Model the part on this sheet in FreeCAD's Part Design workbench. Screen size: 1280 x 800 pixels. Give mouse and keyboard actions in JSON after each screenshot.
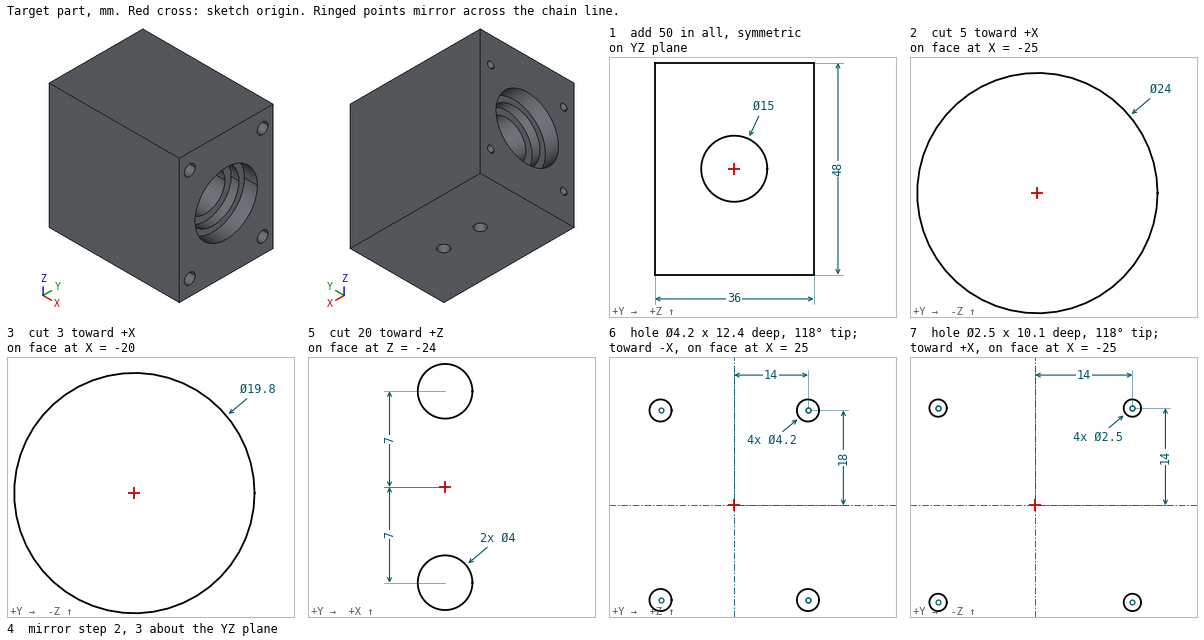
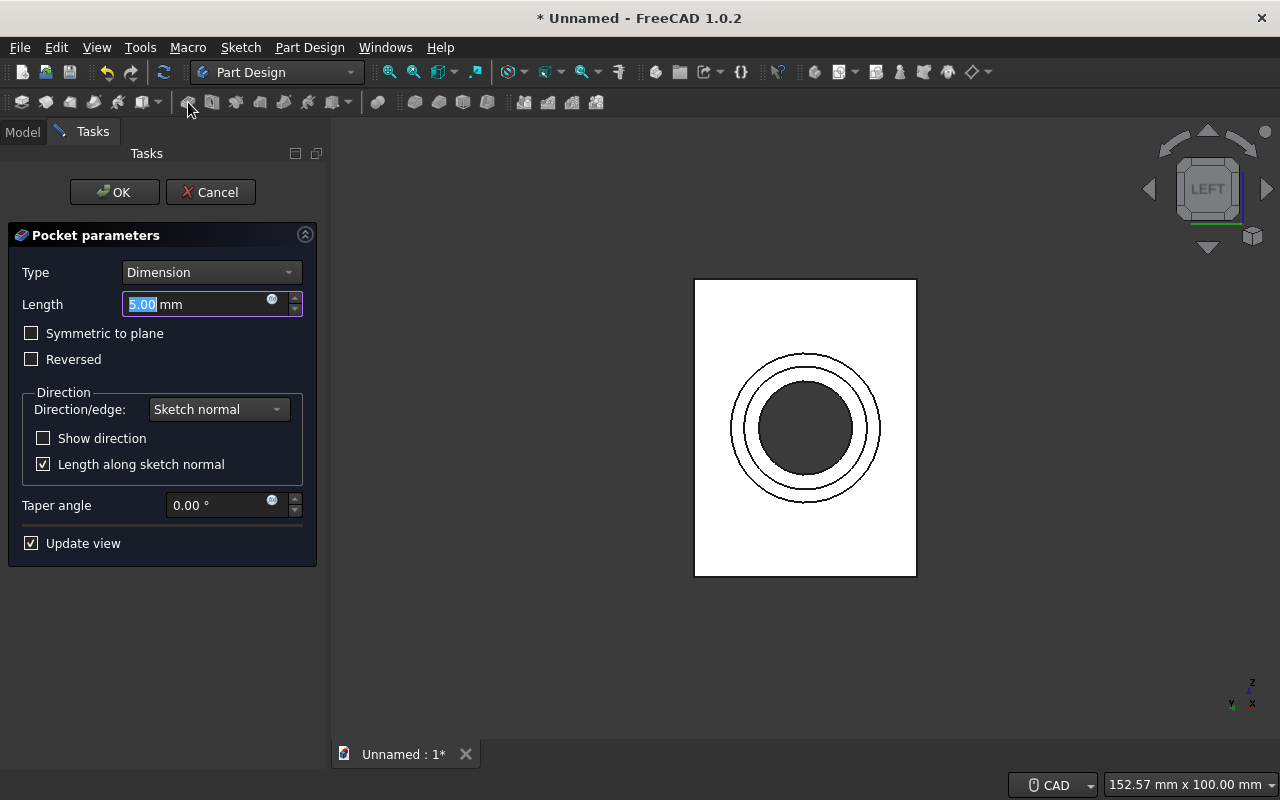
{"action": "type", "text": "3"}
{"action": "key", "text": "Tab"}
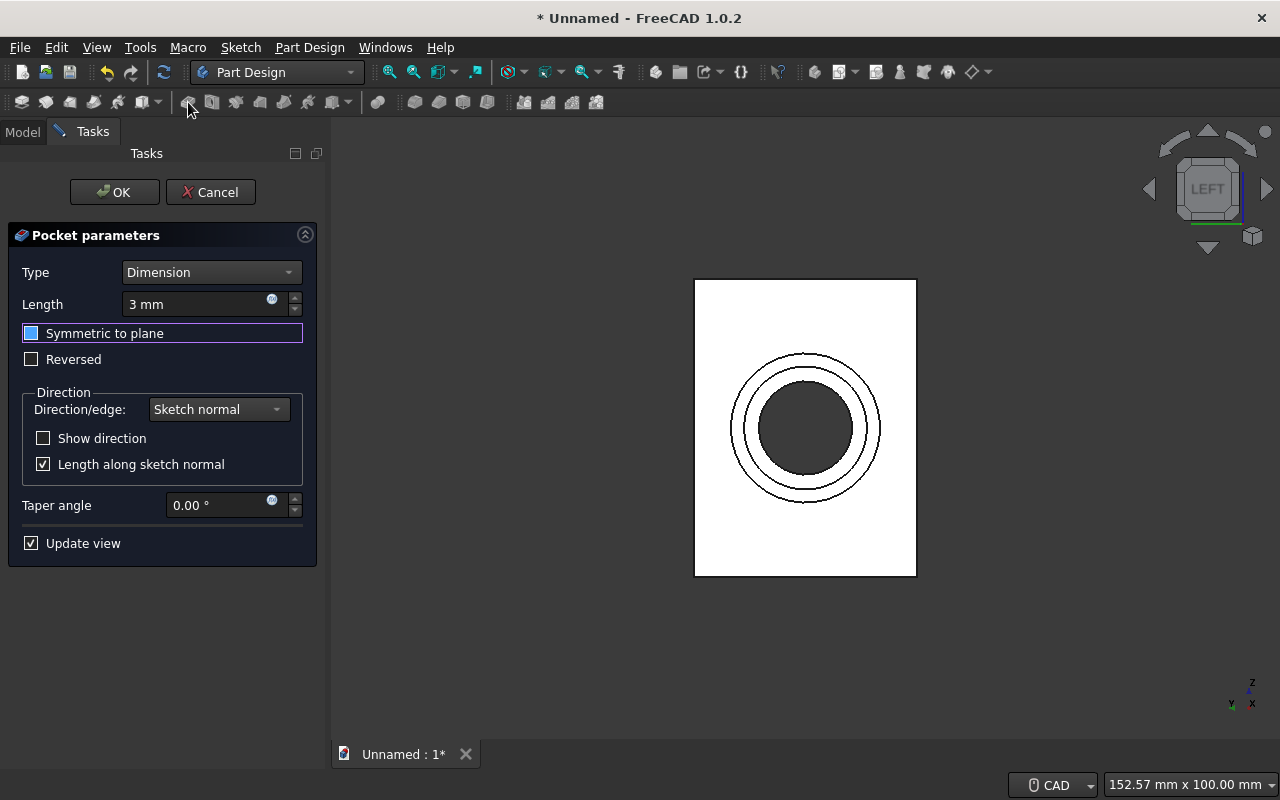
{"action": "left_click", "coordinate": [115, 192]}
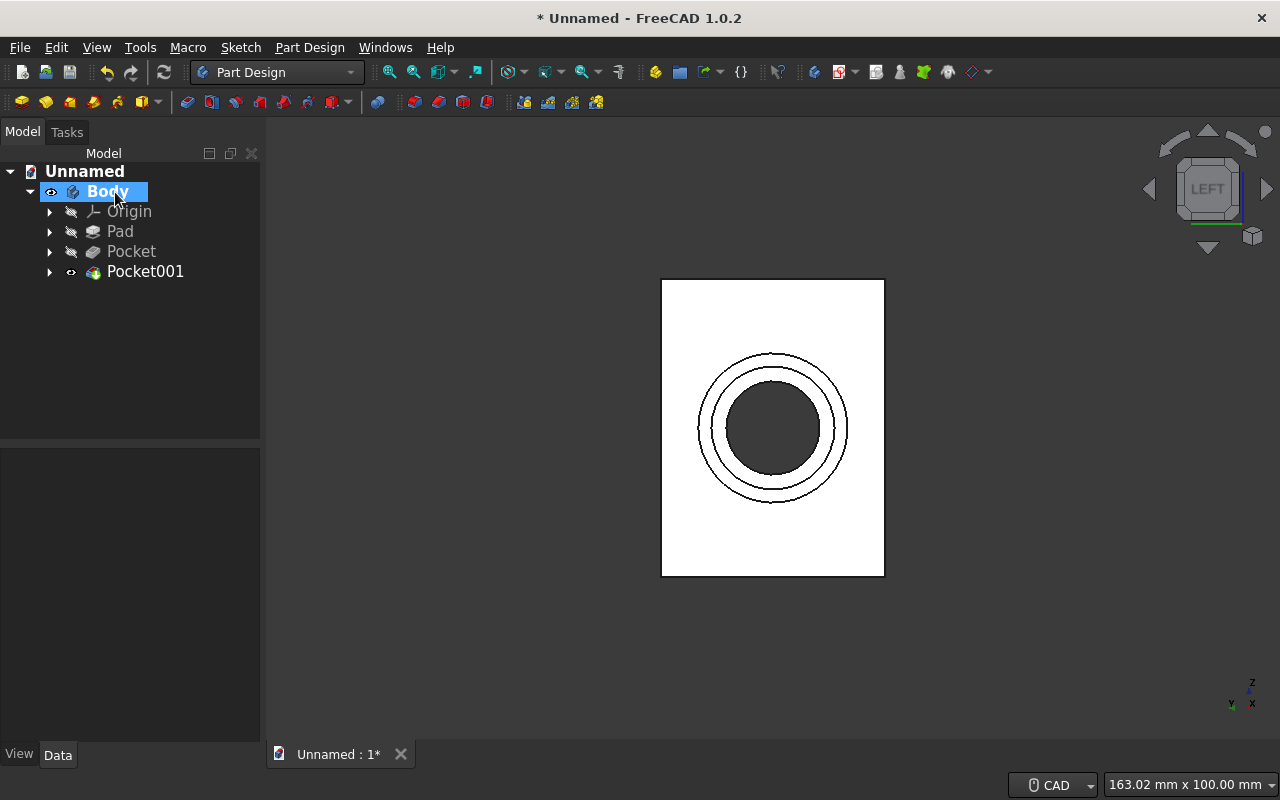
{"action": "left_click", "coordinate": [116, 252]}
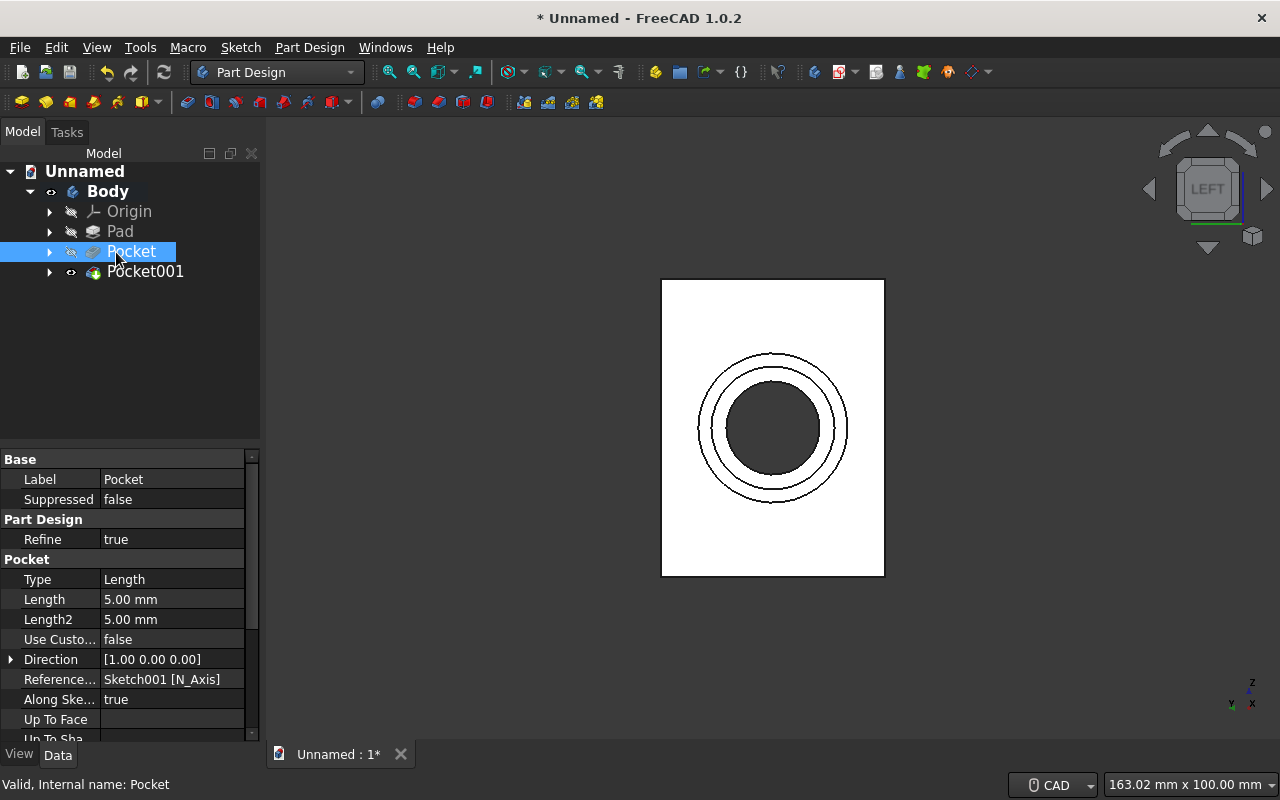
{"action": "left_click", "coordinate": [116, 272], "text": "ctrl"}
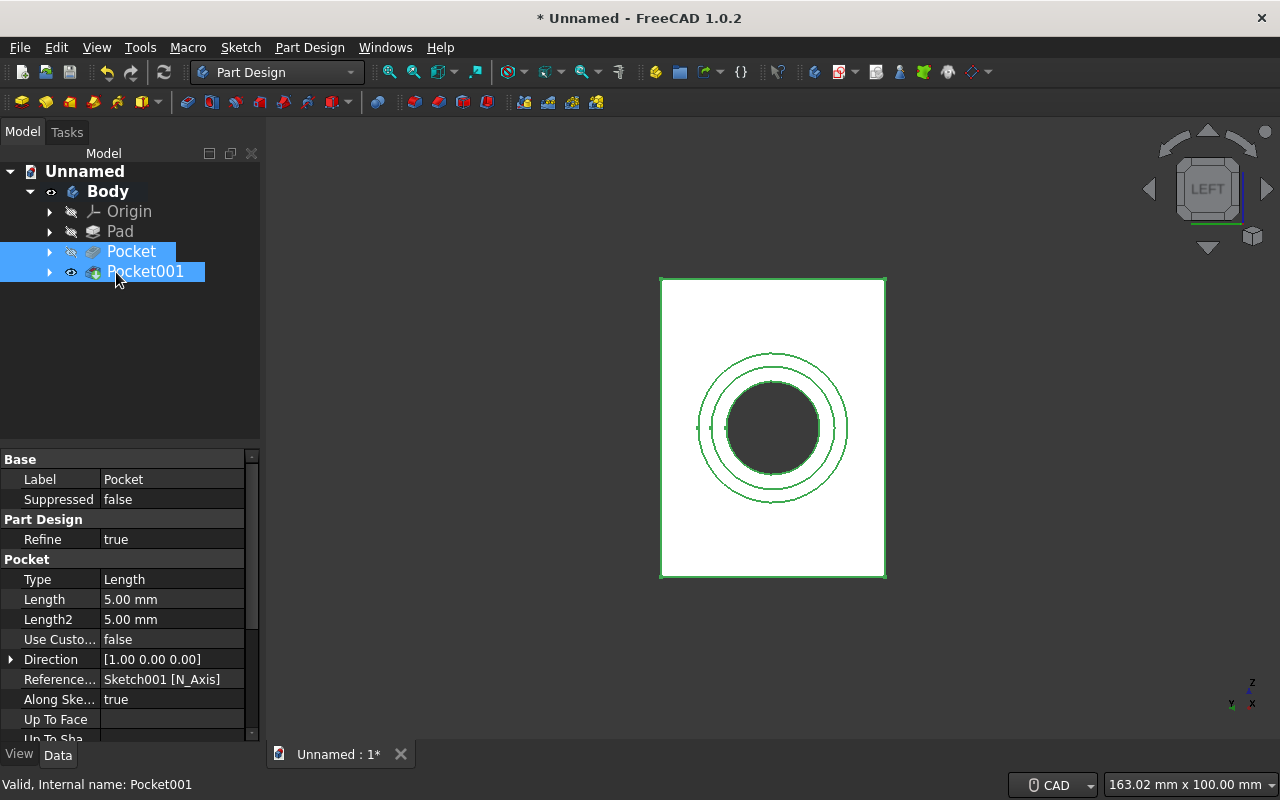
{"action": "left_click", "coordinate": [524, 102]}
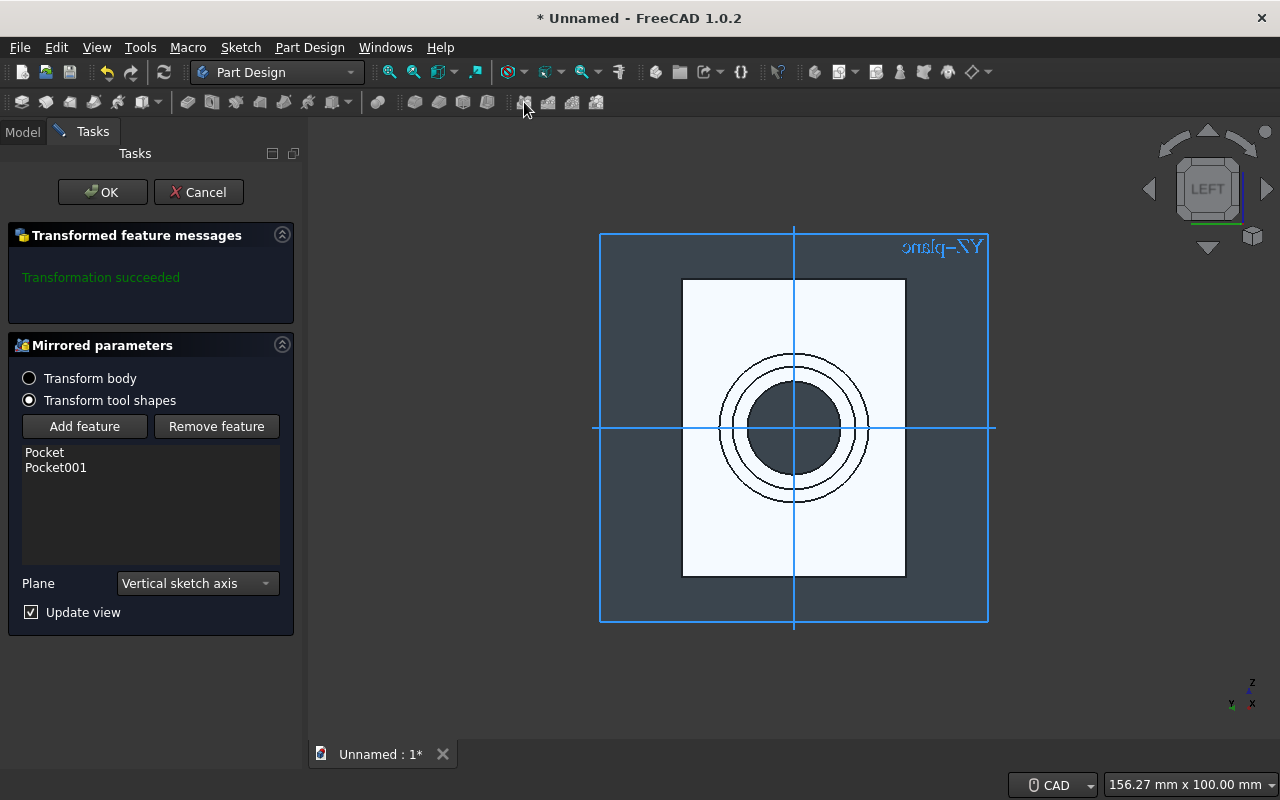
{"action": "left_click", "coordinate": [198, 584]}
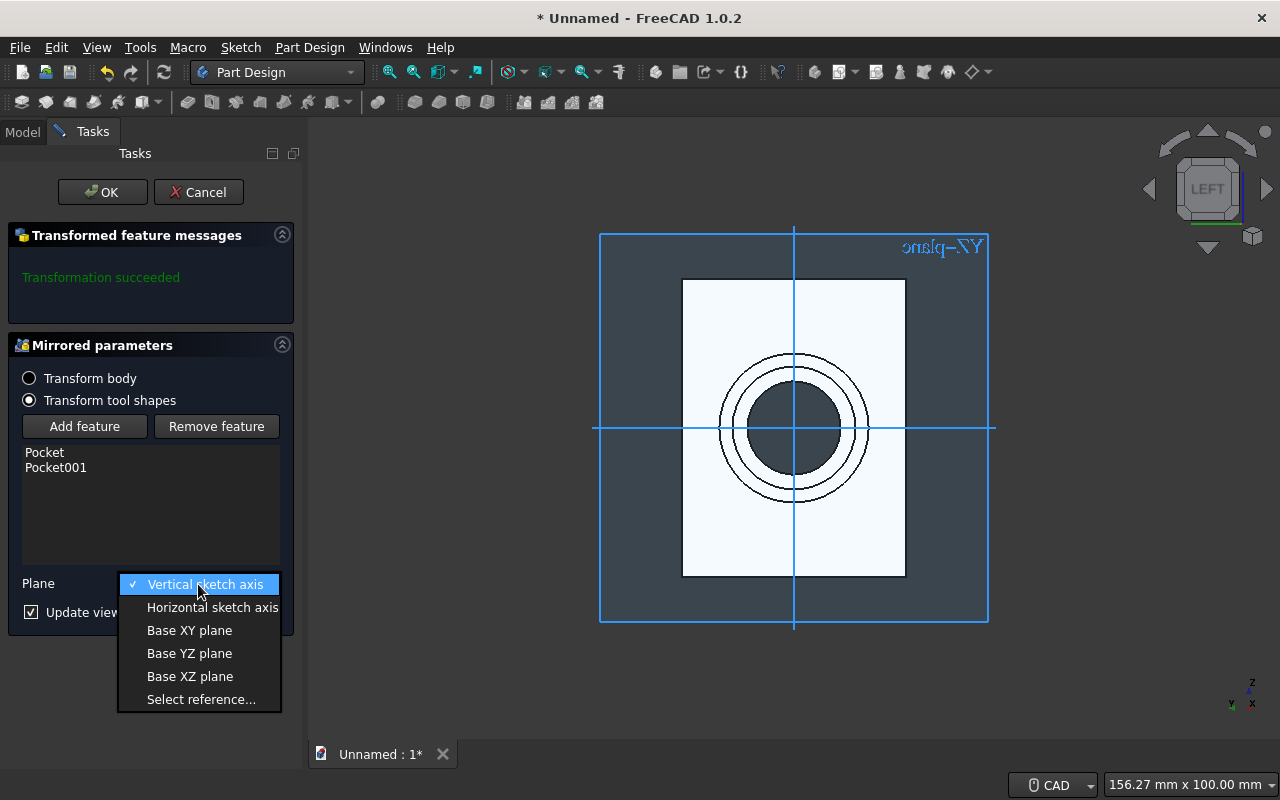
{"action": "left_click", "coordinate": [198, 654]}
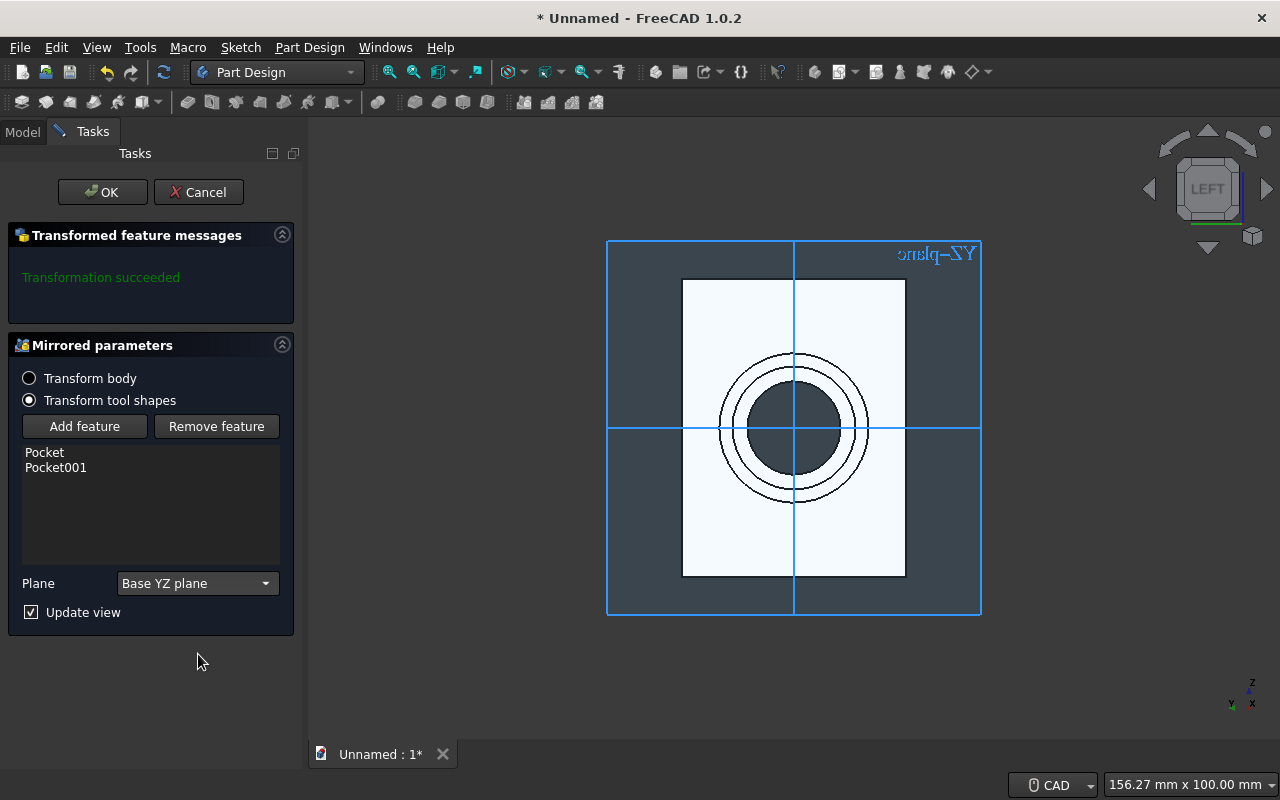
{"action": "left_click", "coordinate": [103, 192]}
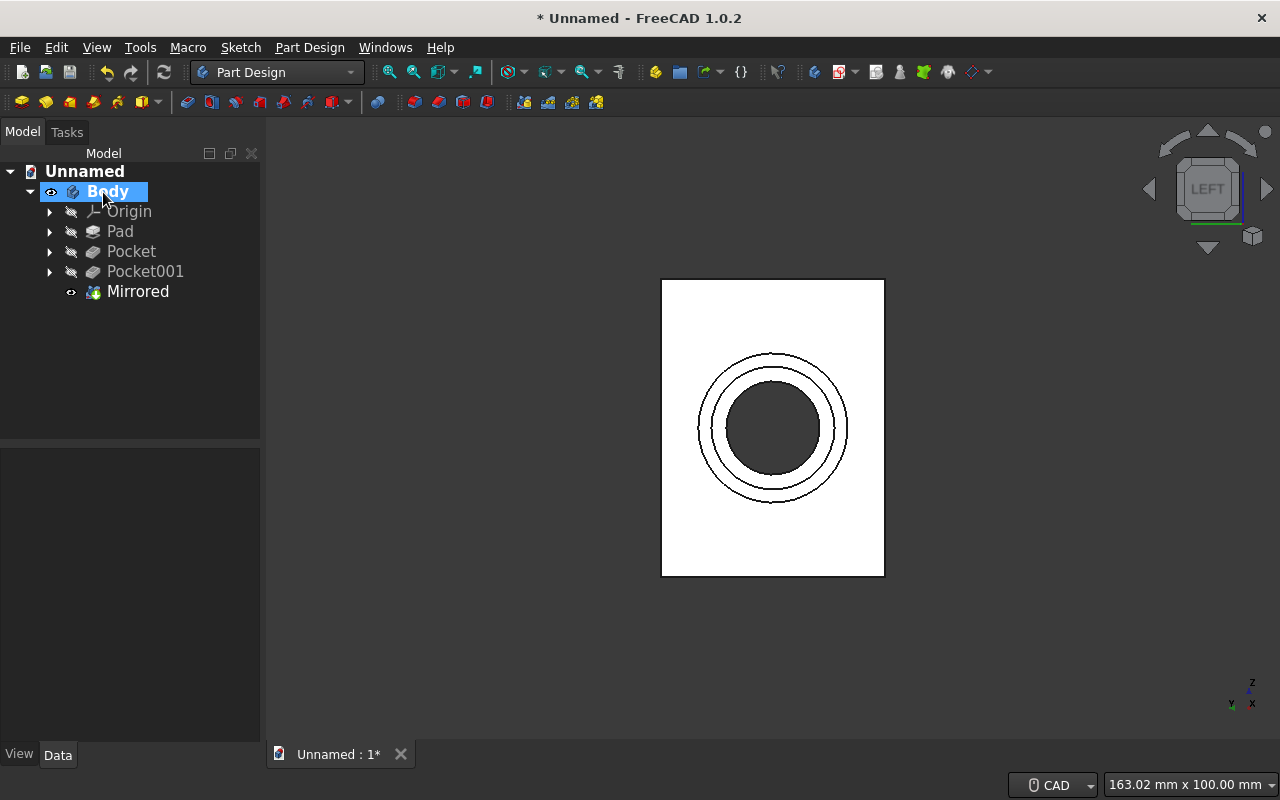
{"action": "key", "text": "5"}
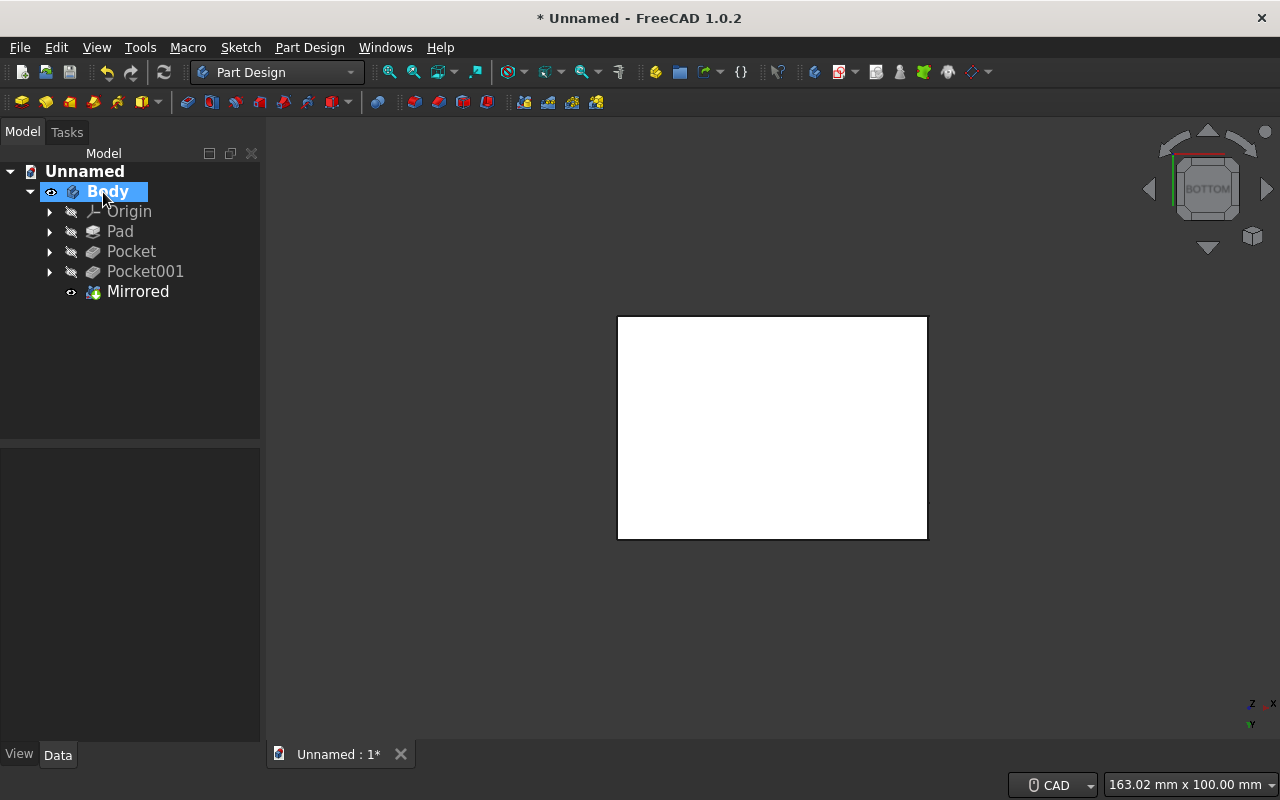
{"action": "left_click", "coordinate": [390, 72]}